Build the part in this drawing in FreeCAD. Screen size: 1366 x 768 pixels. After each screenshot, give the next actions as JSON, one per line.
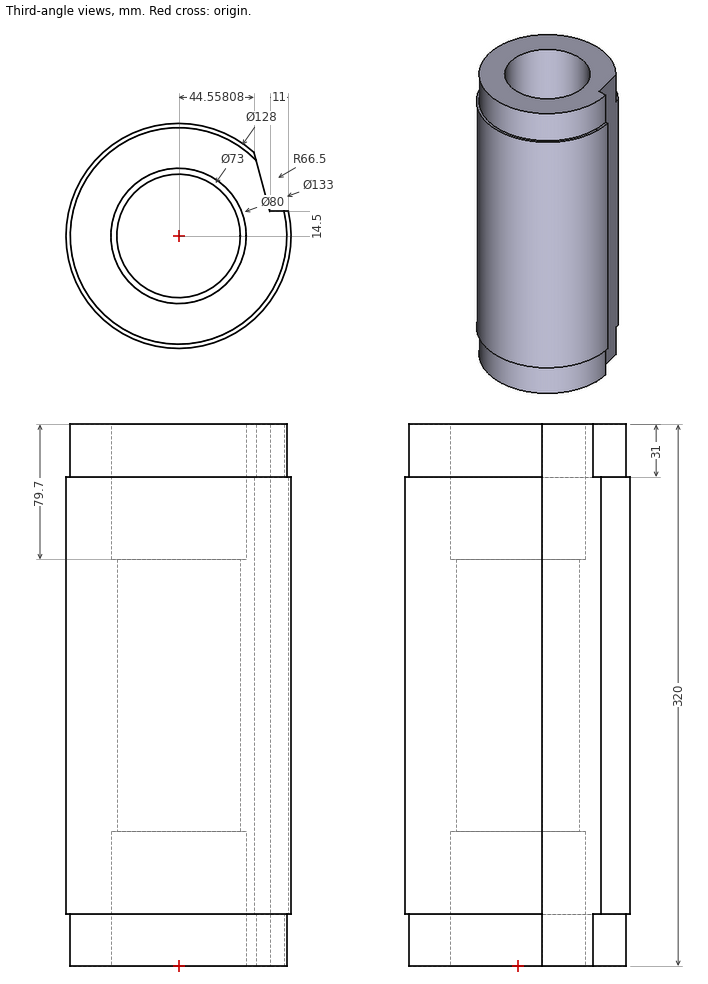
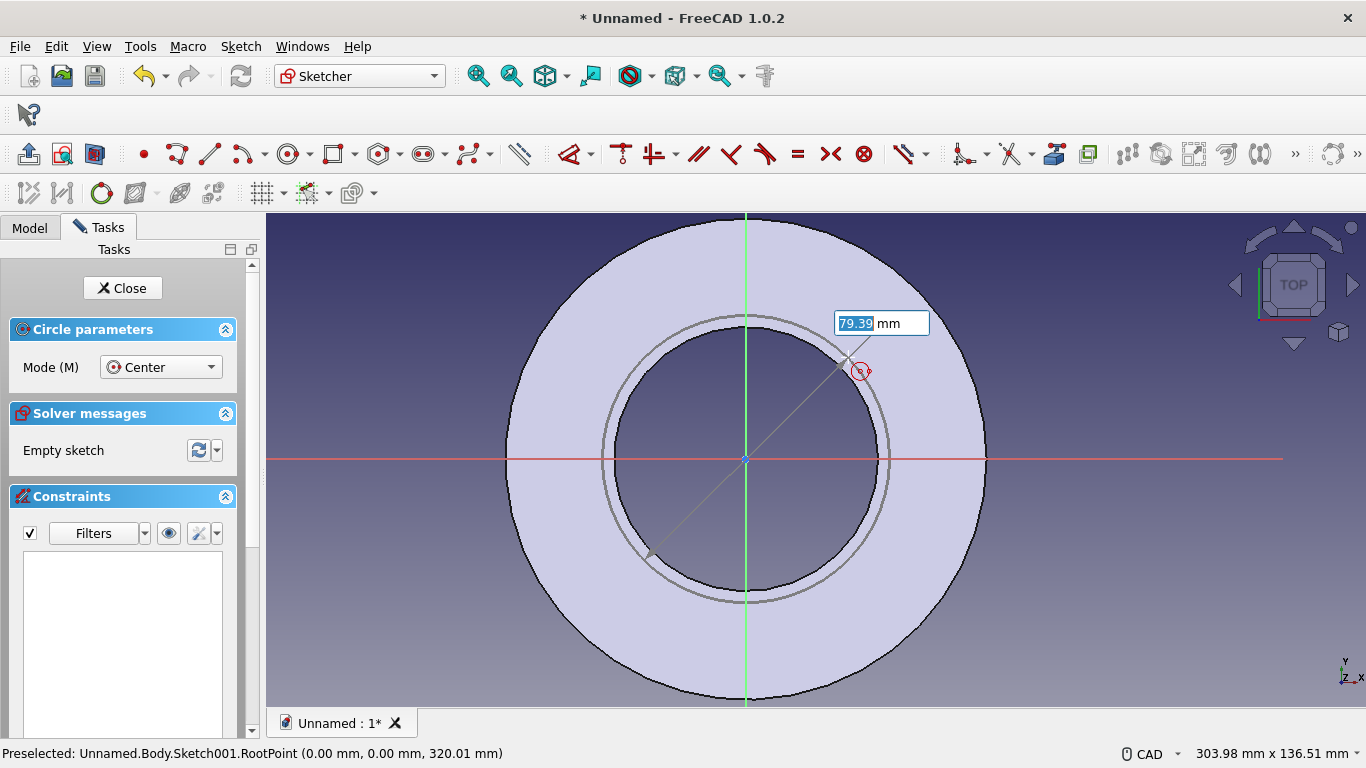
{"action": "type", "text": "80"}
{"action": "key", "text": "Return"}
{"action": "key", "text": "Escape"}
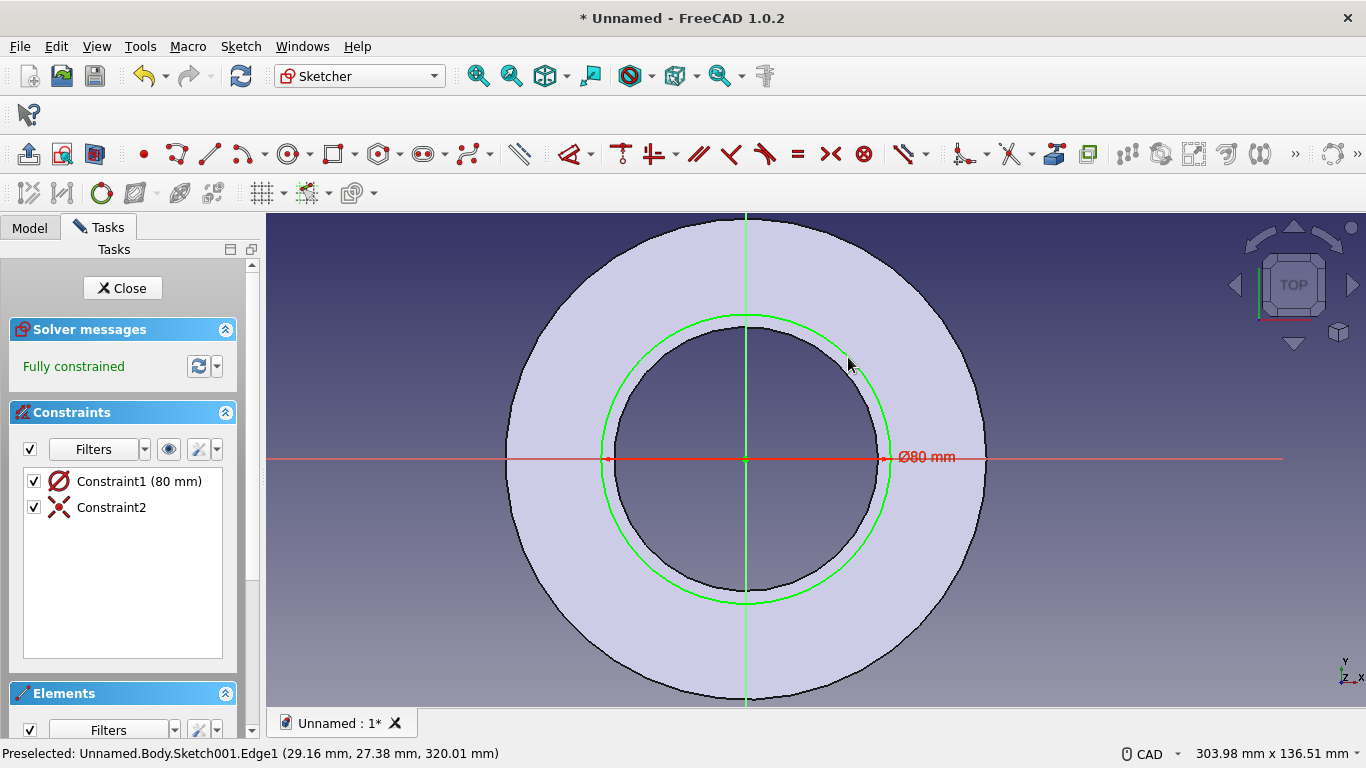
{"action": "left_click", "coordinate": [123, 288]}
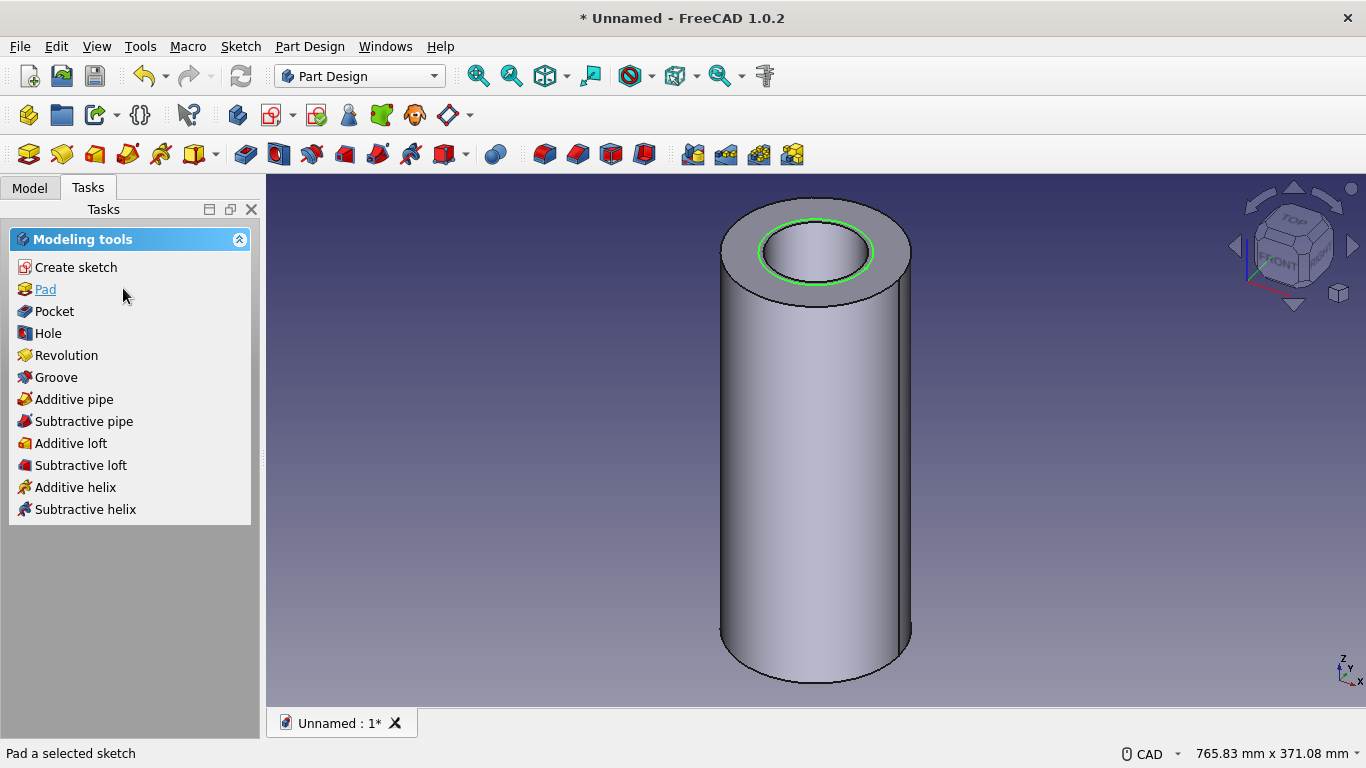
{"action": "left_click", "coordinate": [246, 154]}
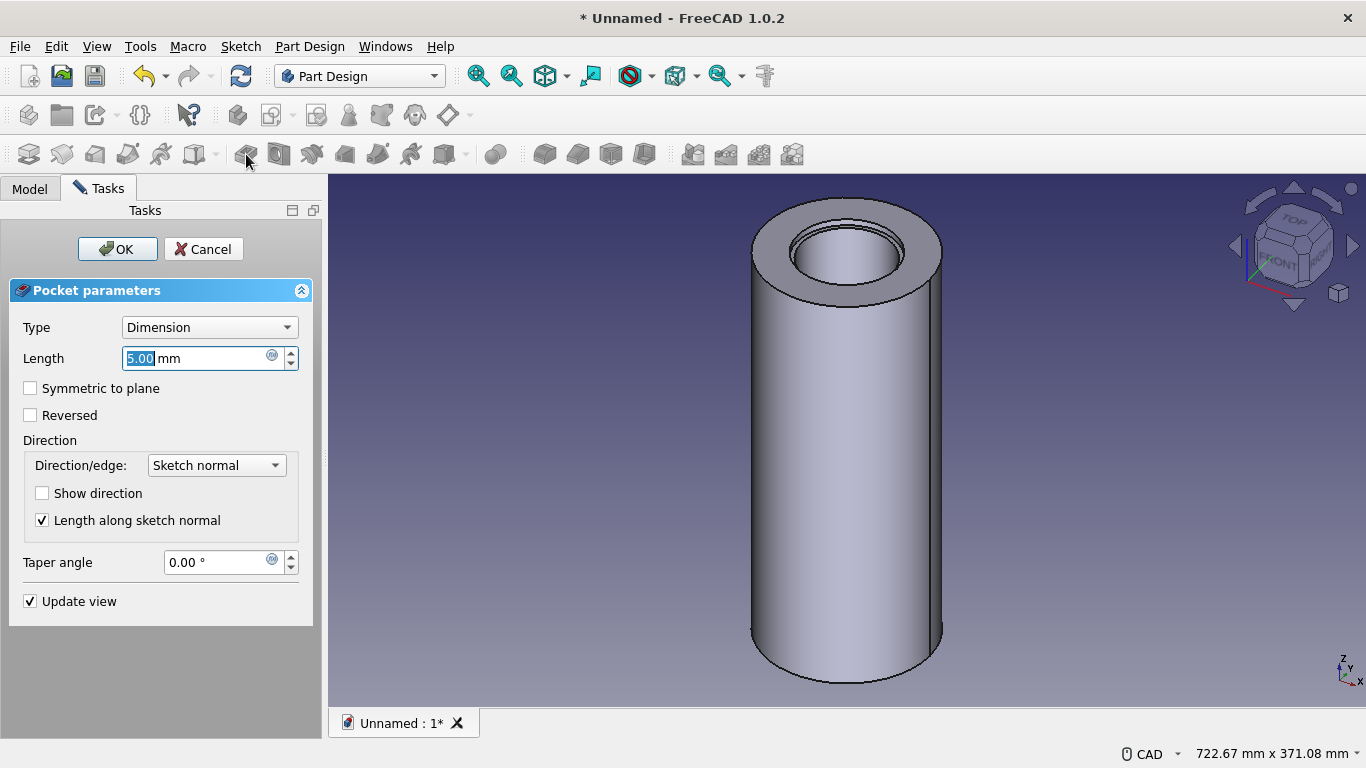
{"action": "type", "text": "79.7"}
{"action": "key", "text": "Tab"}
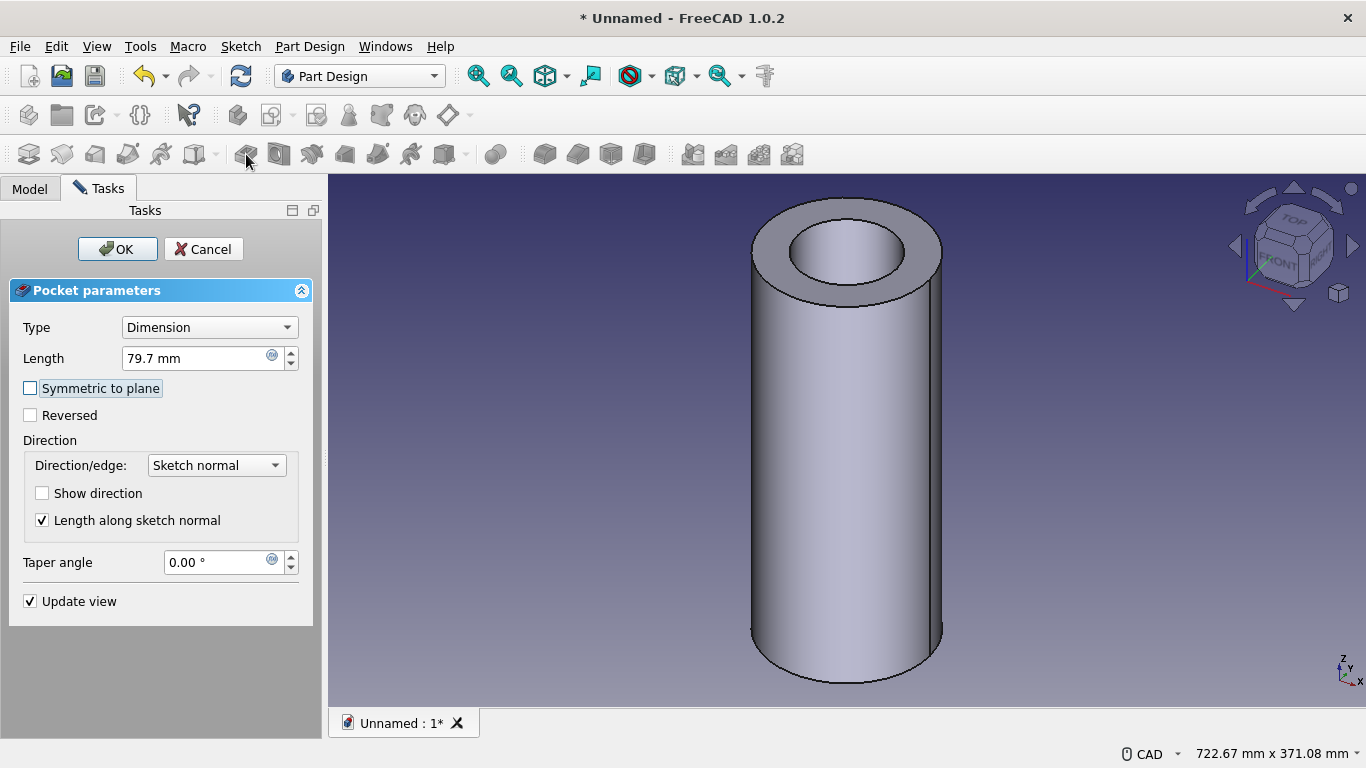
{"action": "left_click", "coordinate": [118, 249]}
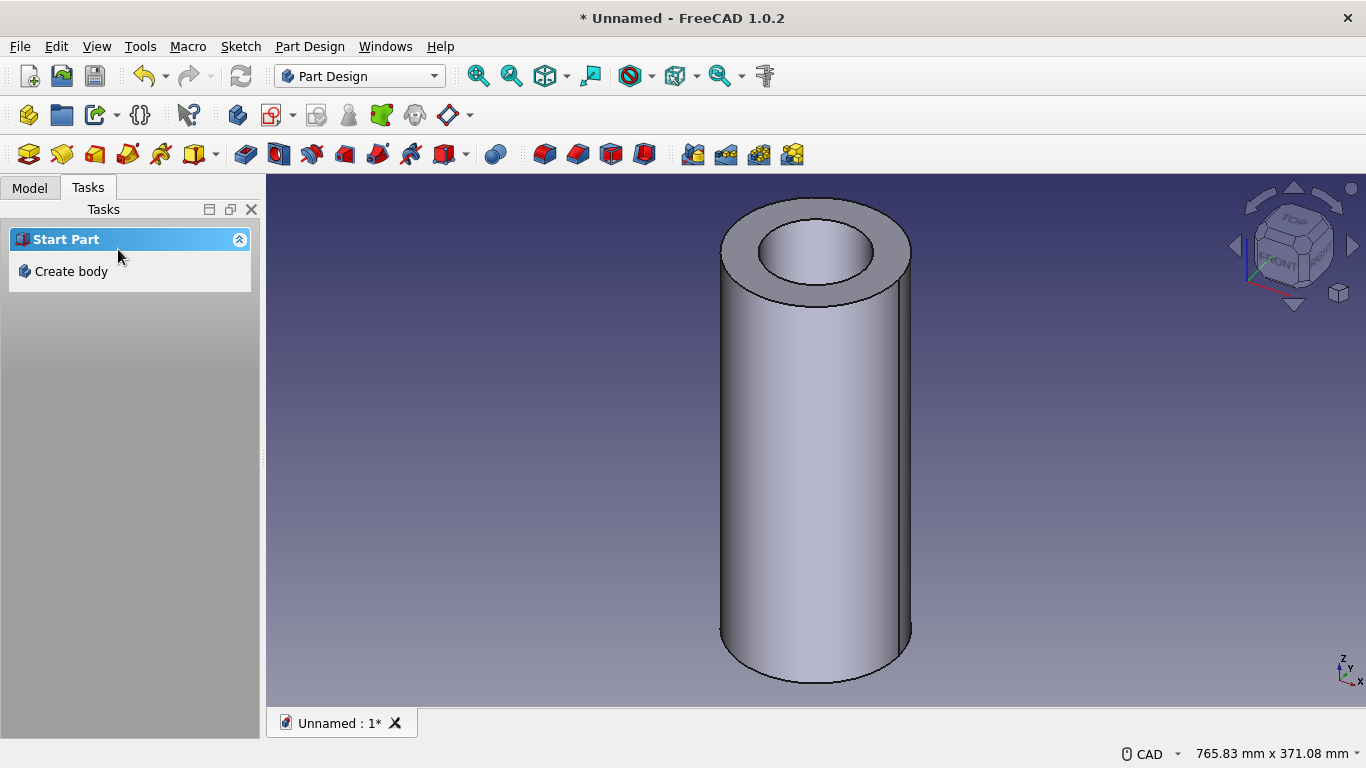
{"action": "left_click", "coordinate": [30, 188]}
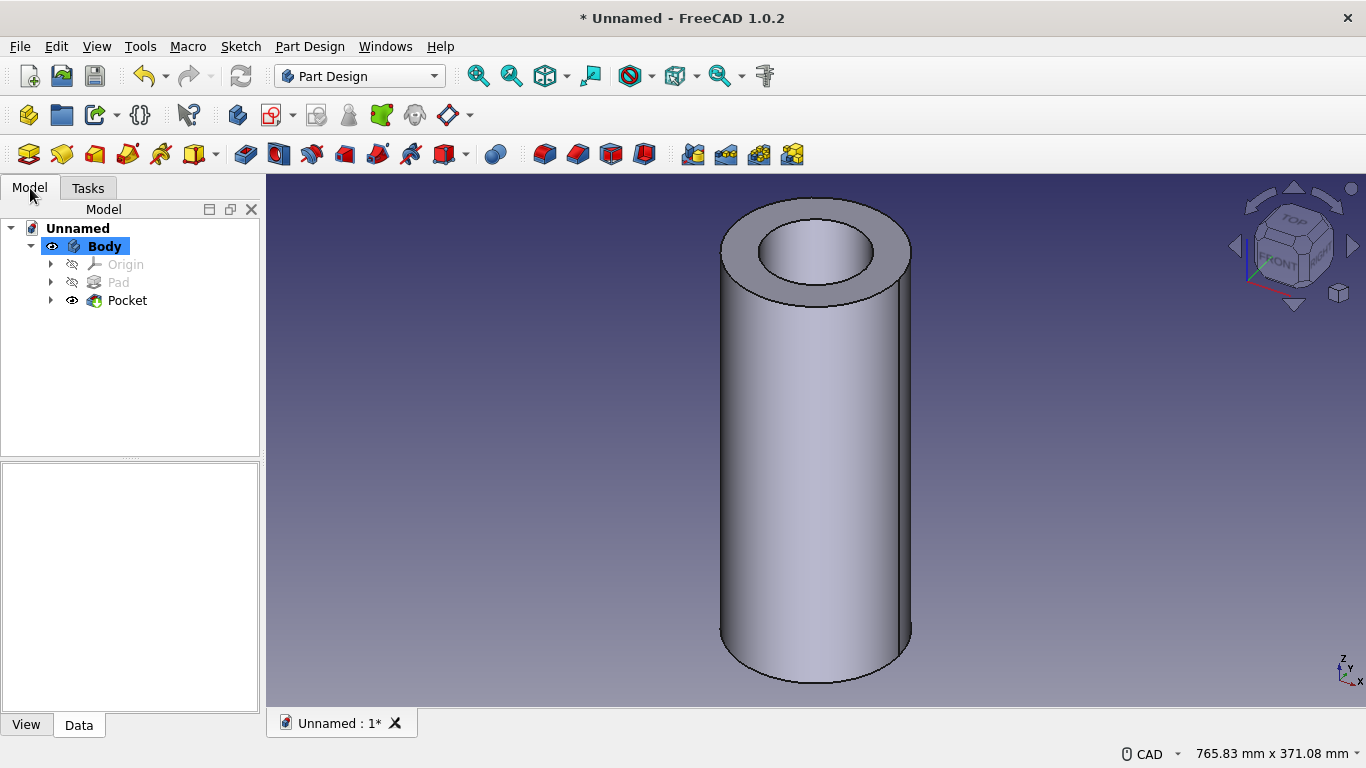
{"action": "left_click", "coordinate": [51, 264]}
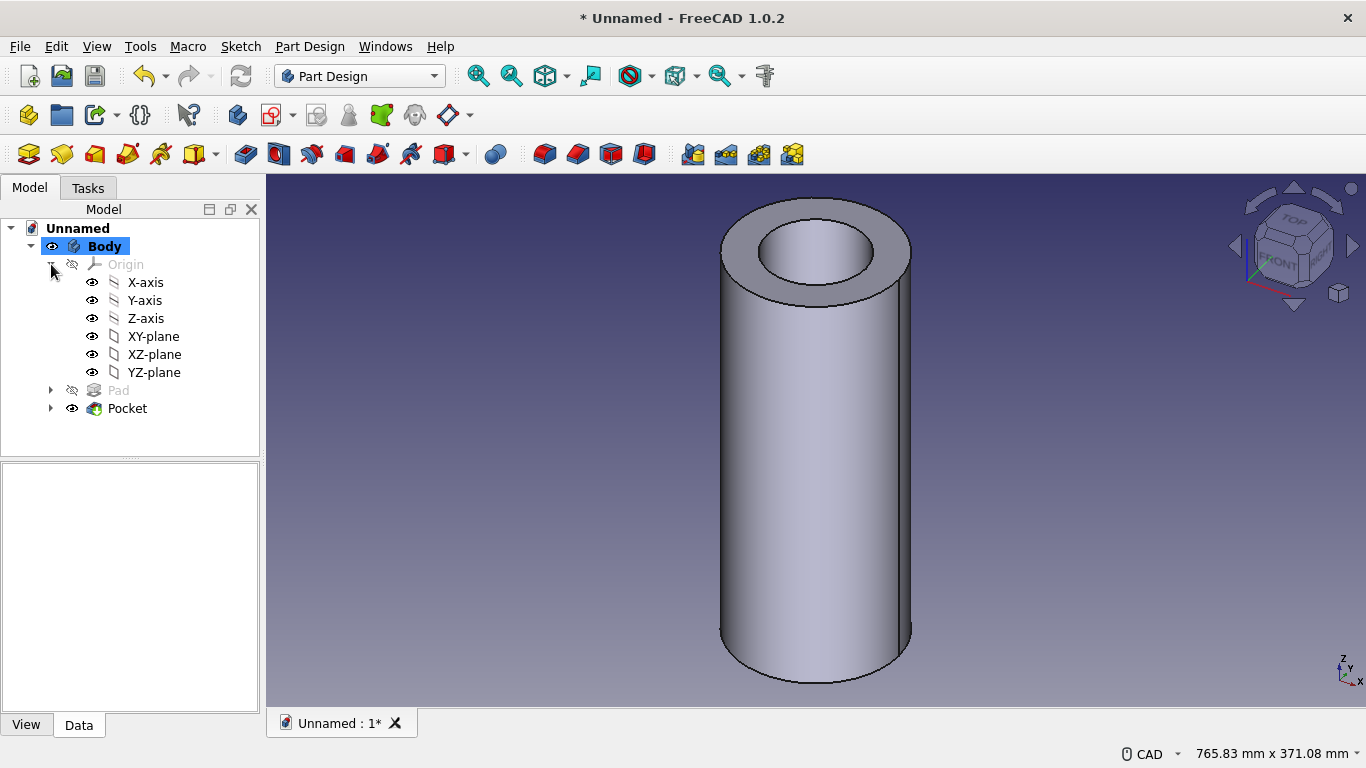
{"action": "left_click", "coordinate": [137, 336]}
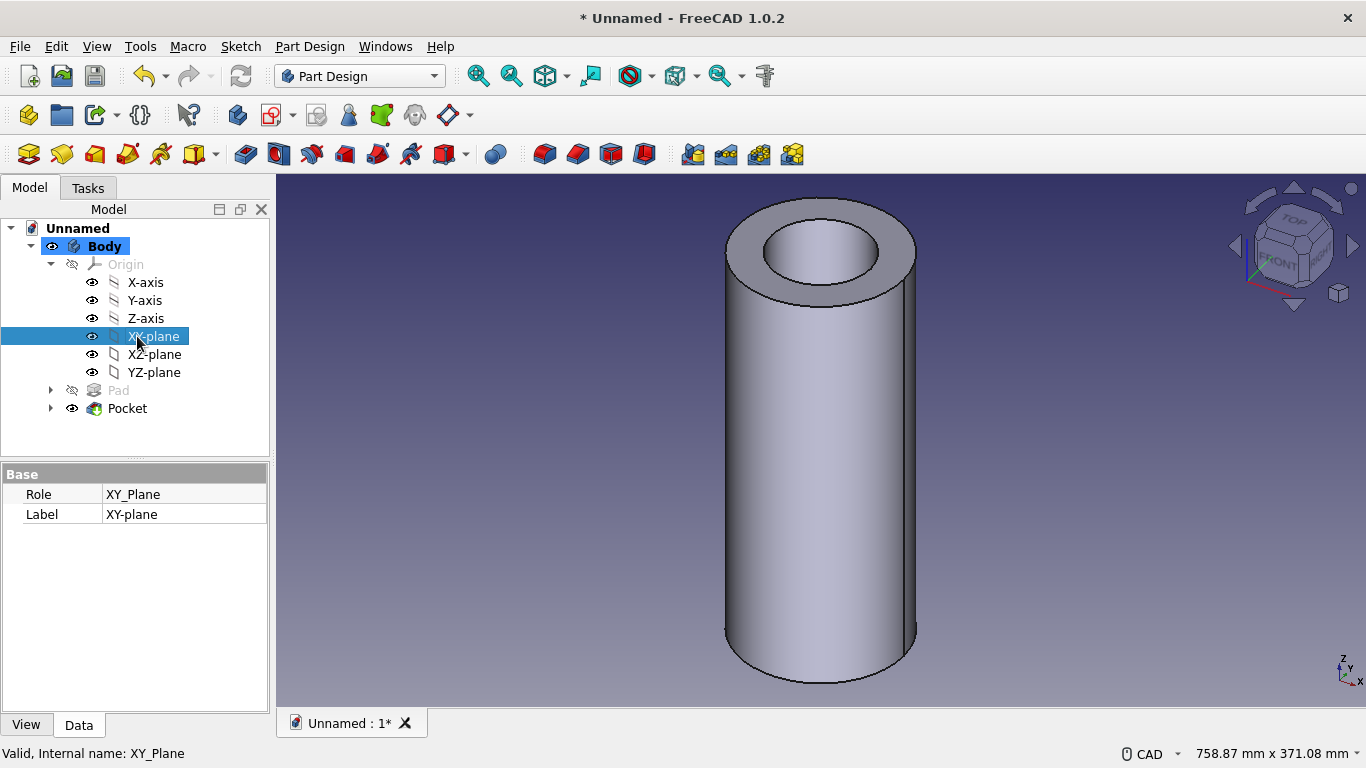
{"action": "left_click", "coordinate": [448, 116]}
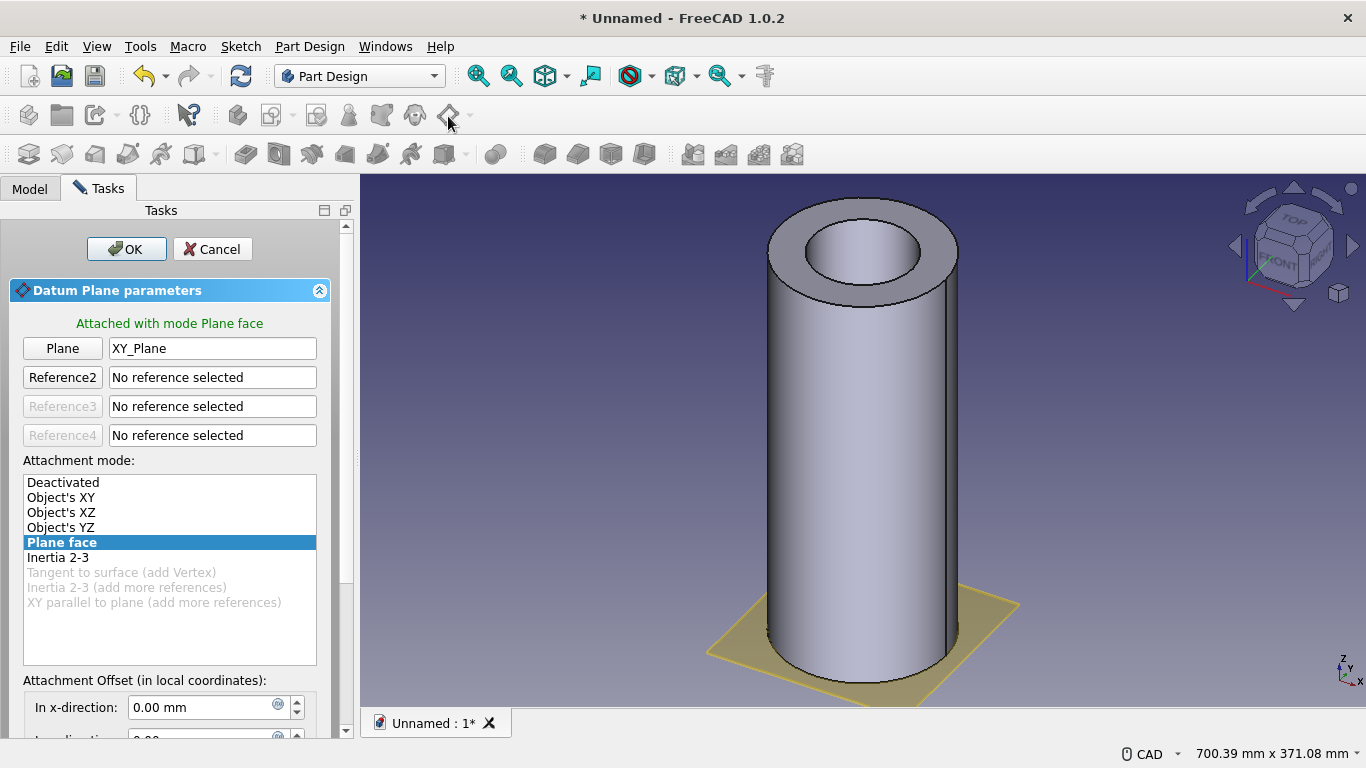
{"action": "scroll", "coordinate": [346, 479], "scroll_direction": "down", "scroll_amount": 2}